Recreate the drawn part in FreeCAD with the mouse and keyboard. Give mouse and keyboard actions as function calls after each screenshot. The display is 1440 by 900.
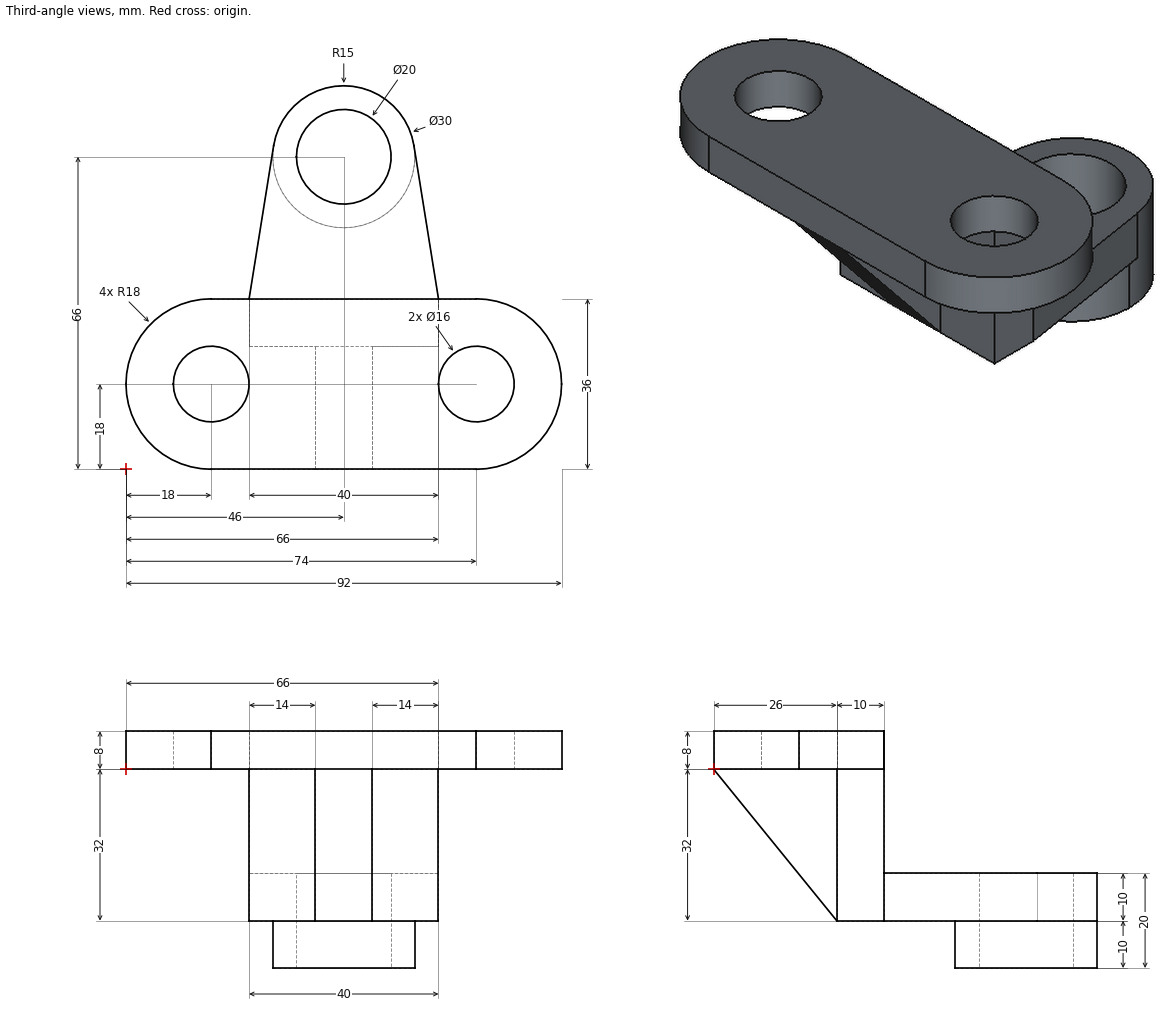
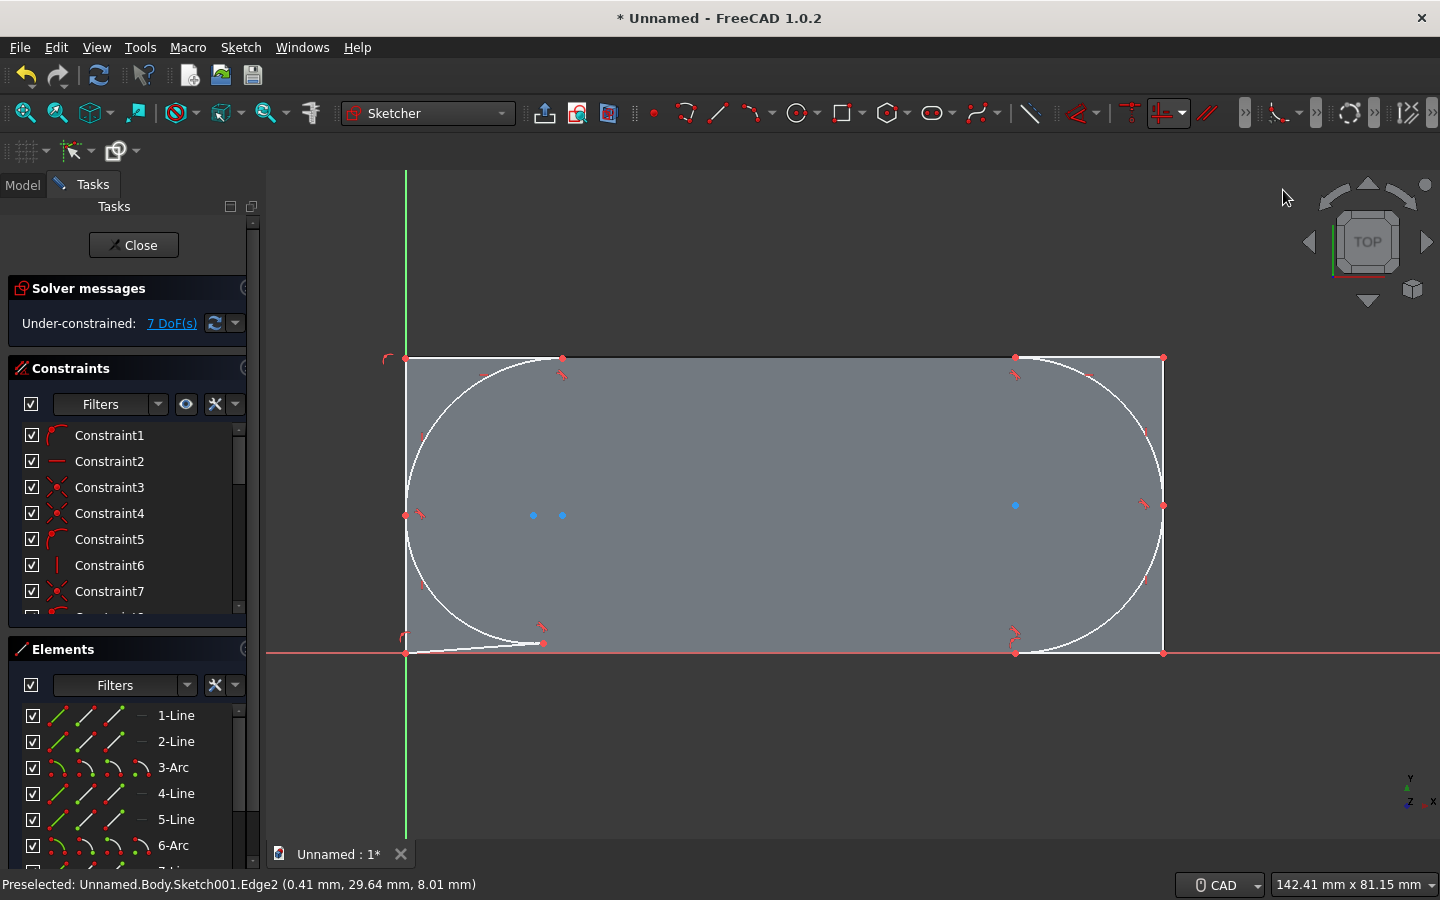
click(447, 650)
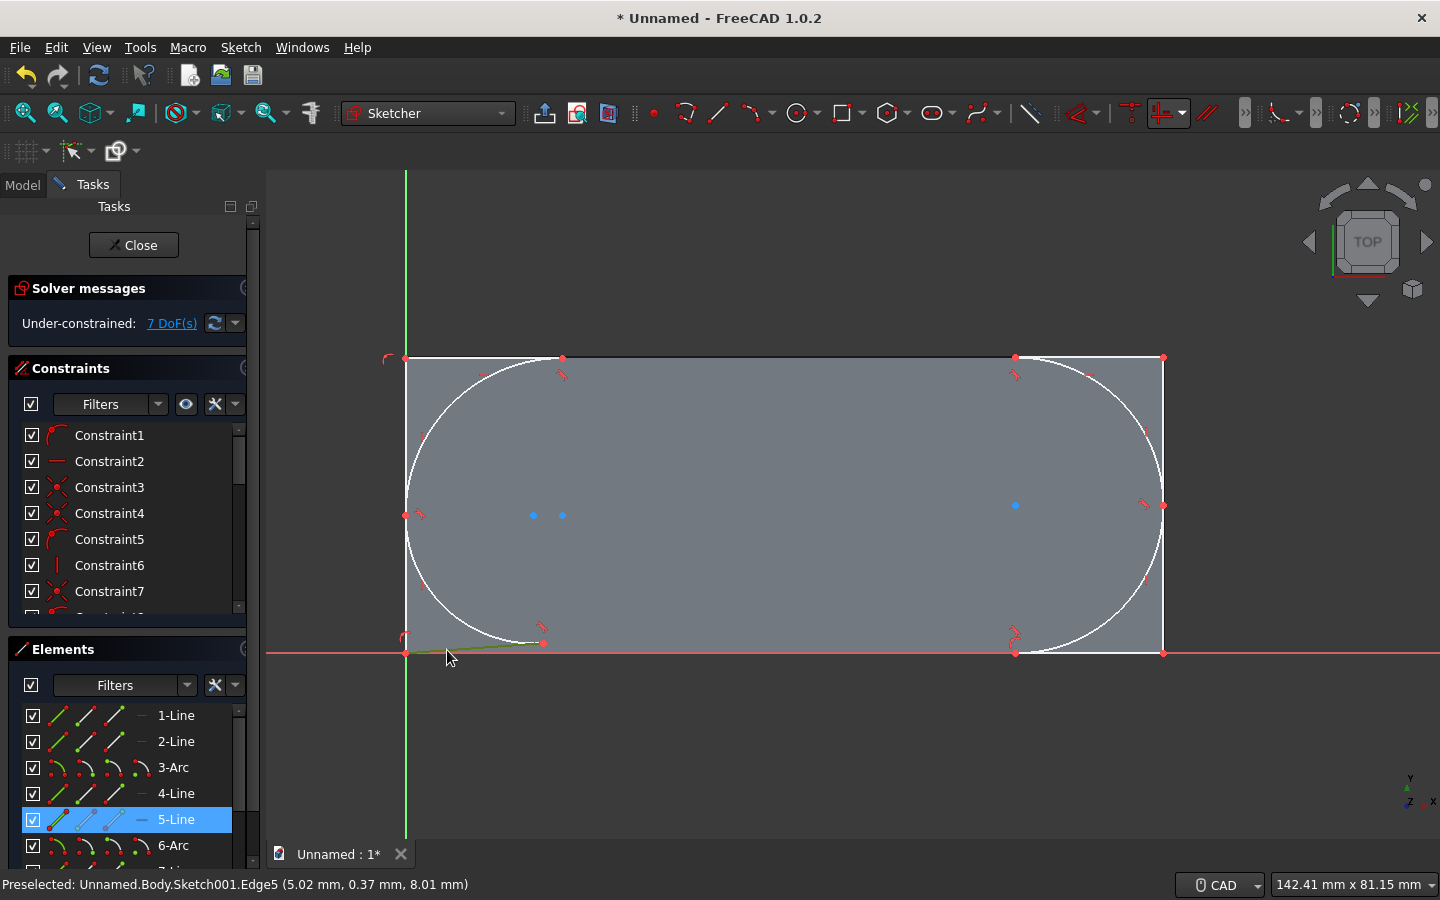
click(1184, 114)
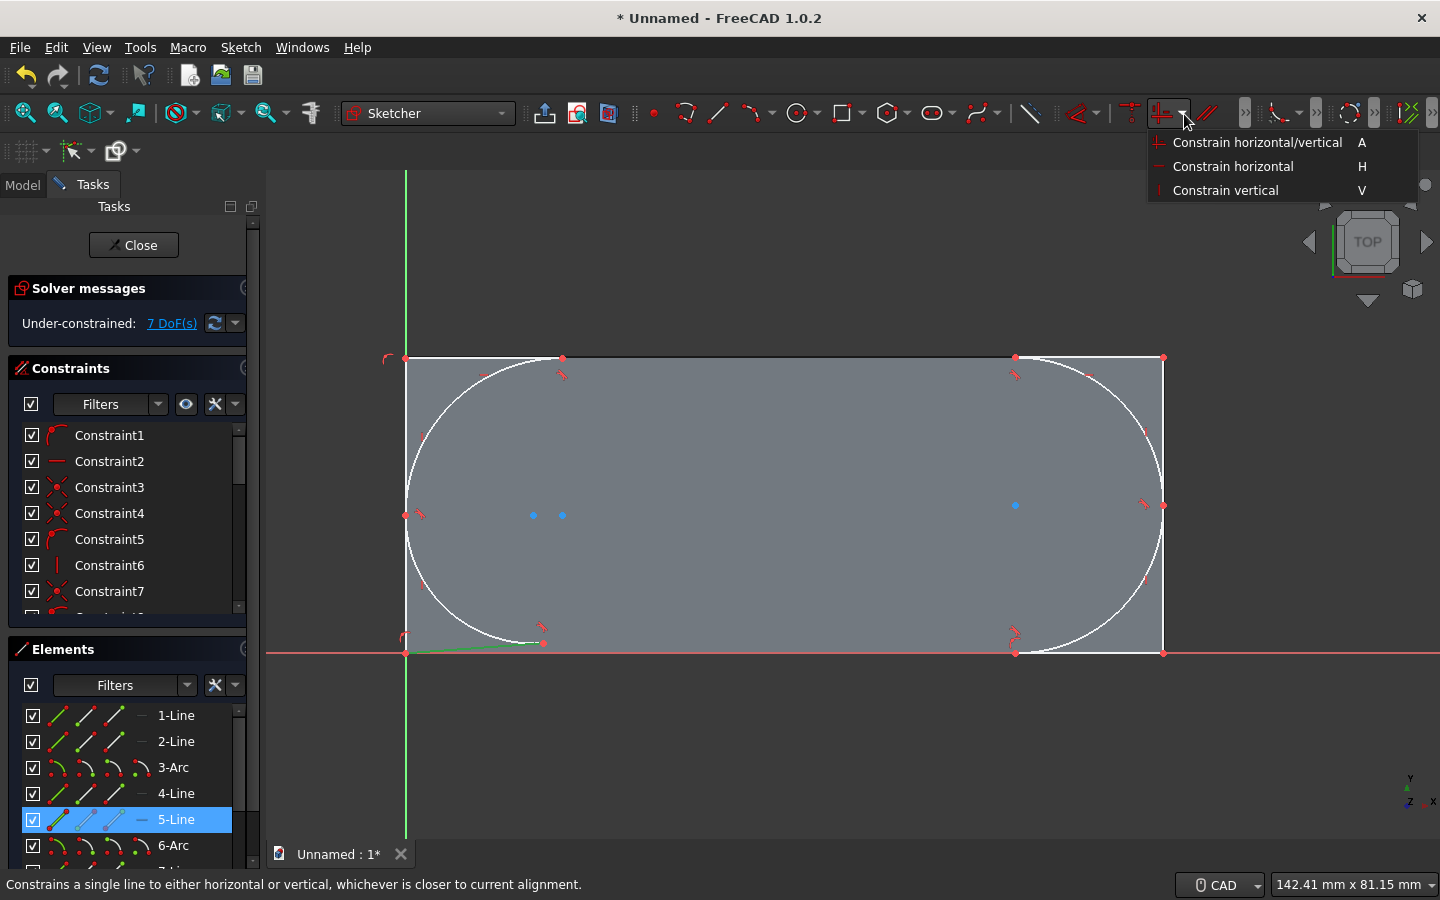
click(1283, 166)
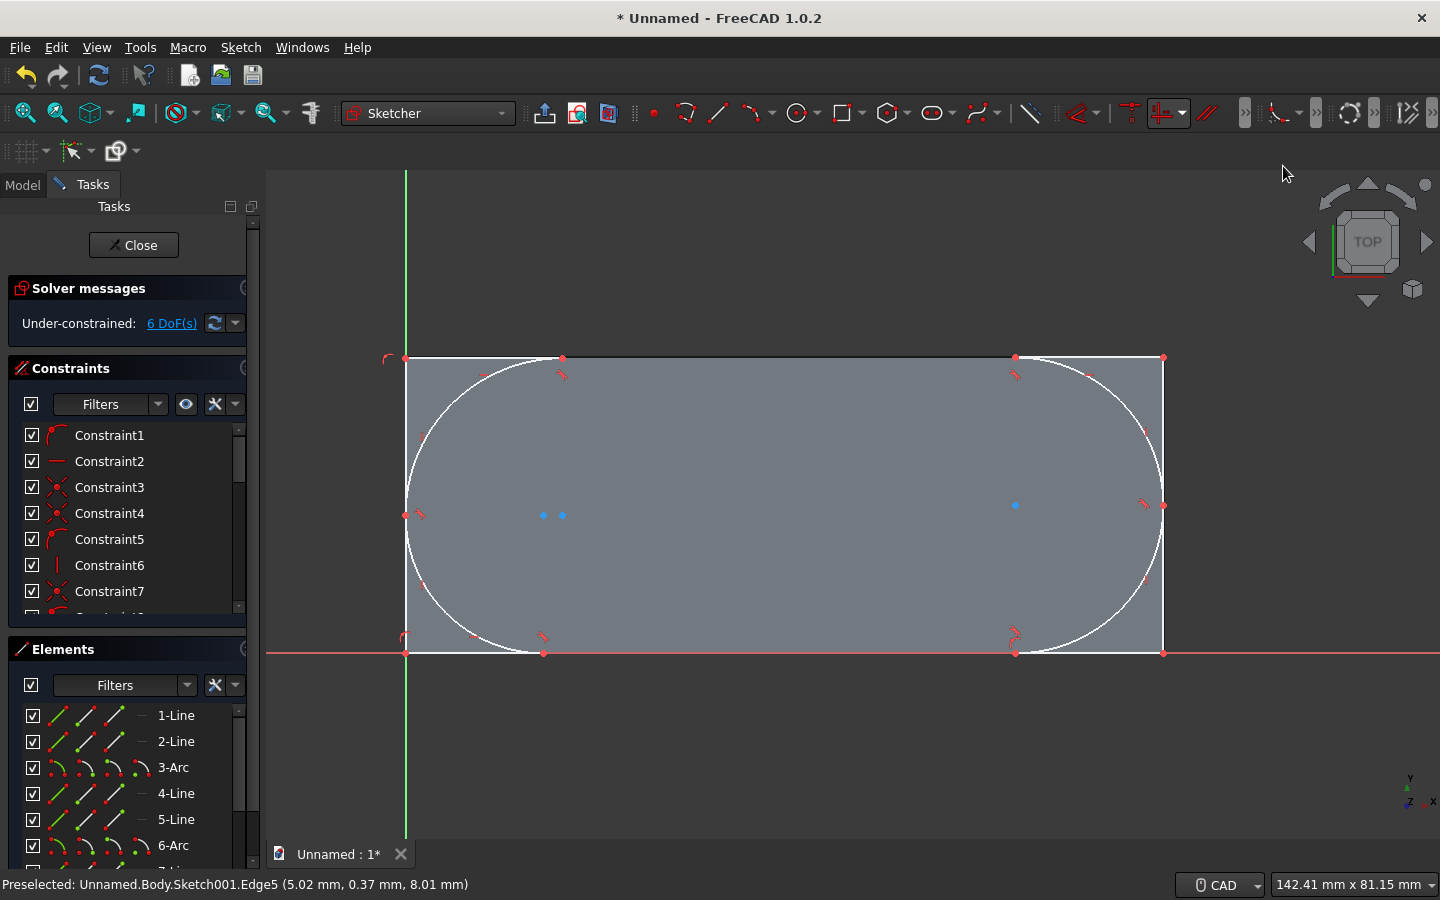
click(1119, 653)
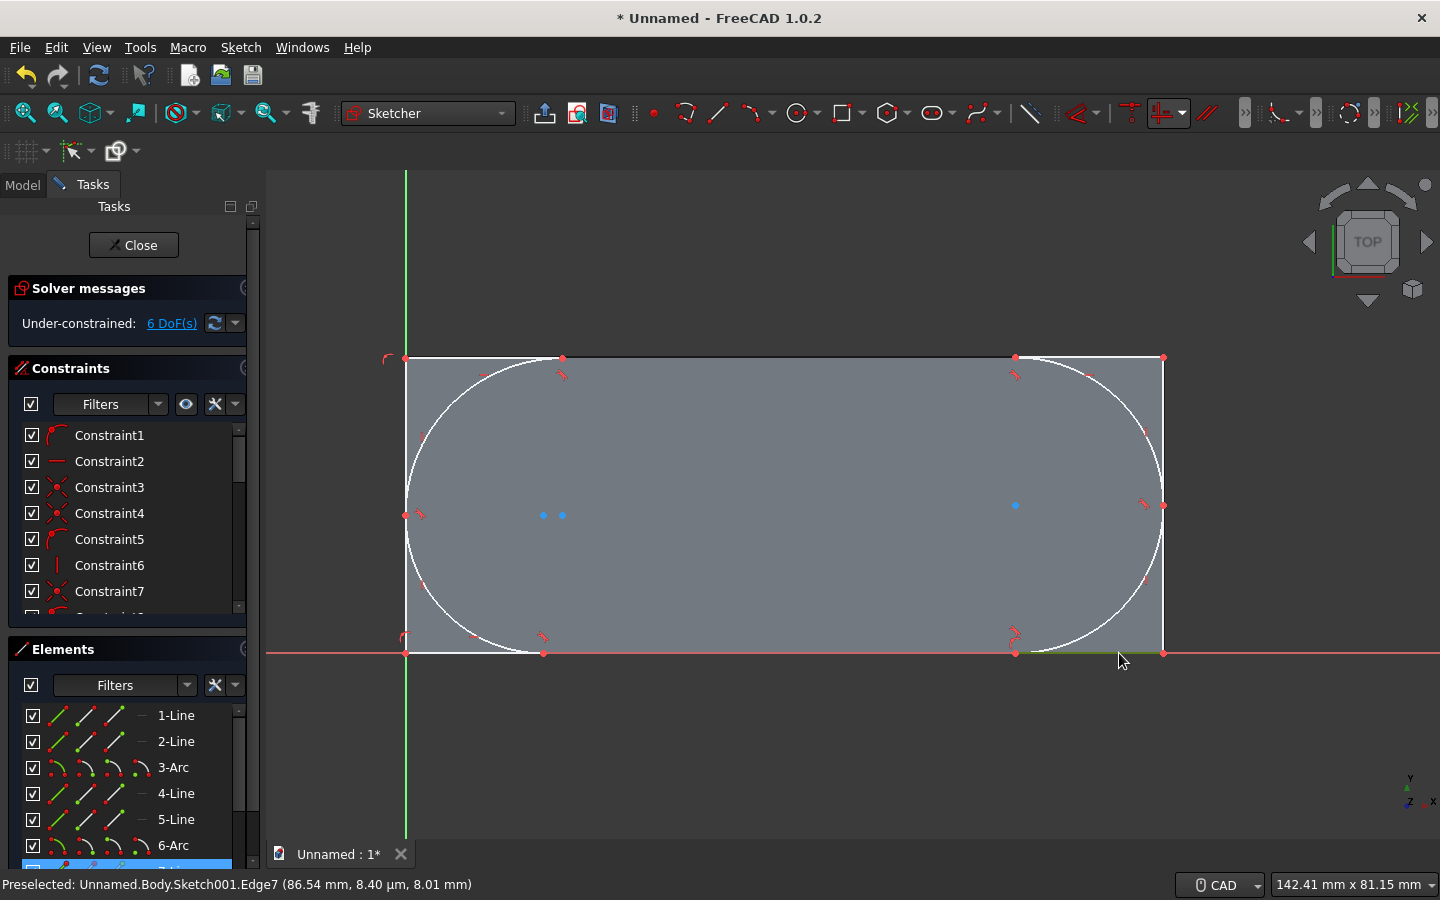
click(1184, 114)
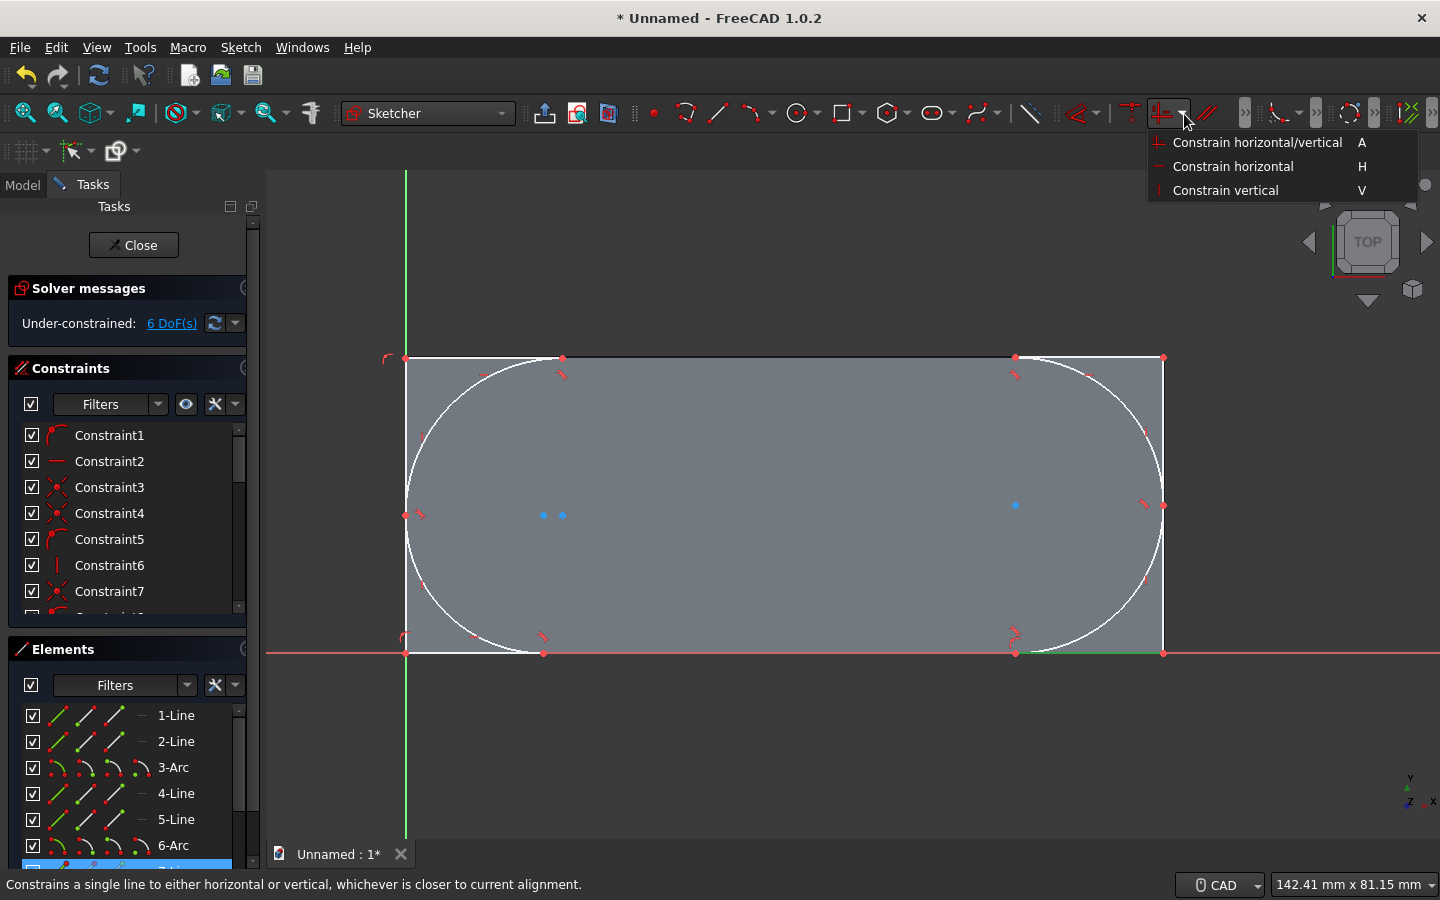
click(1283, 166)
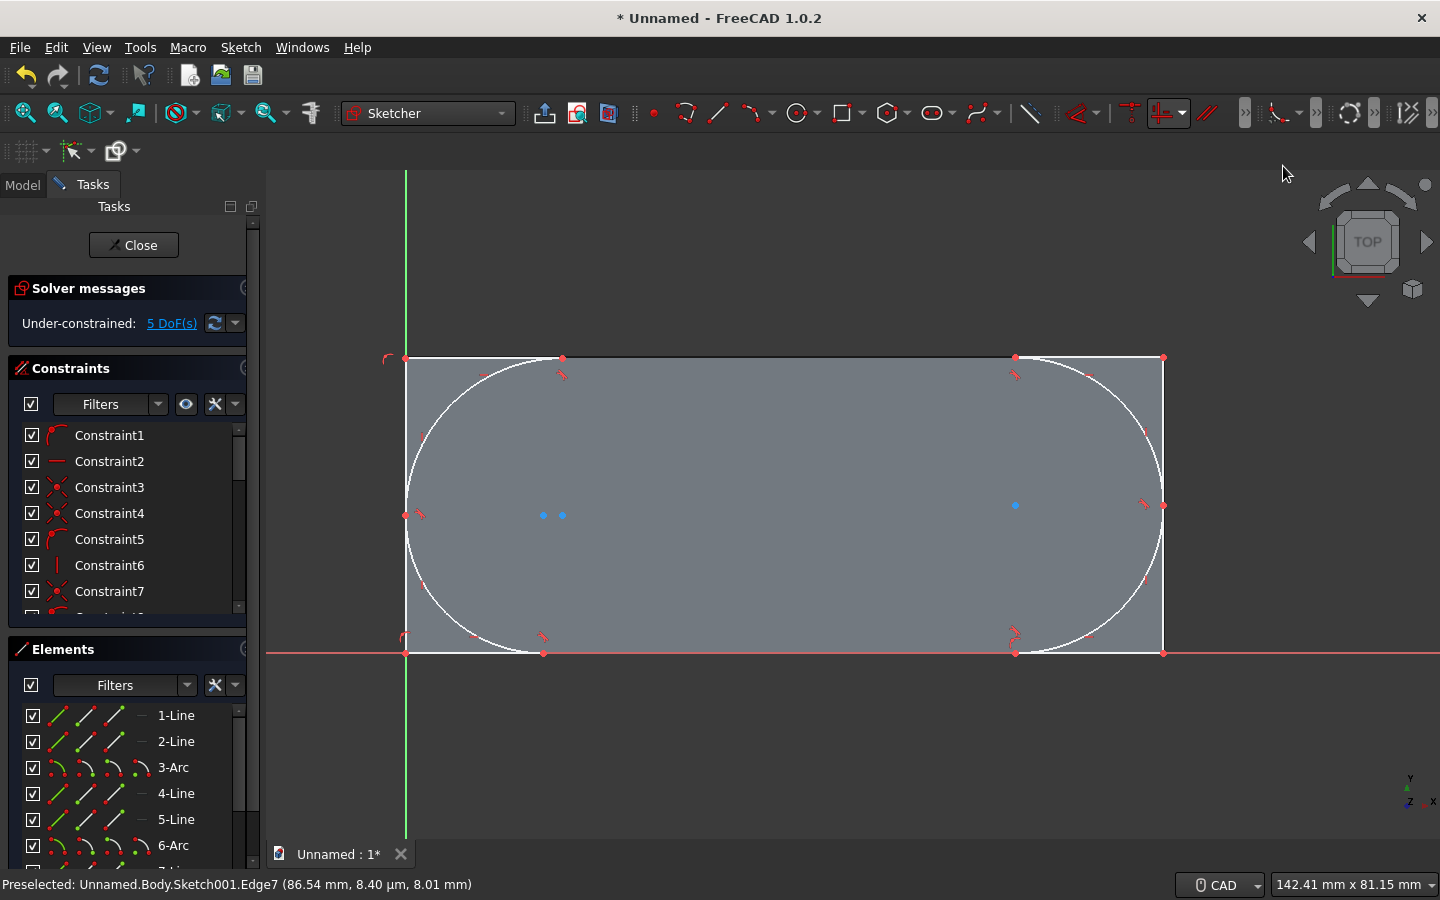
click(491, 375)